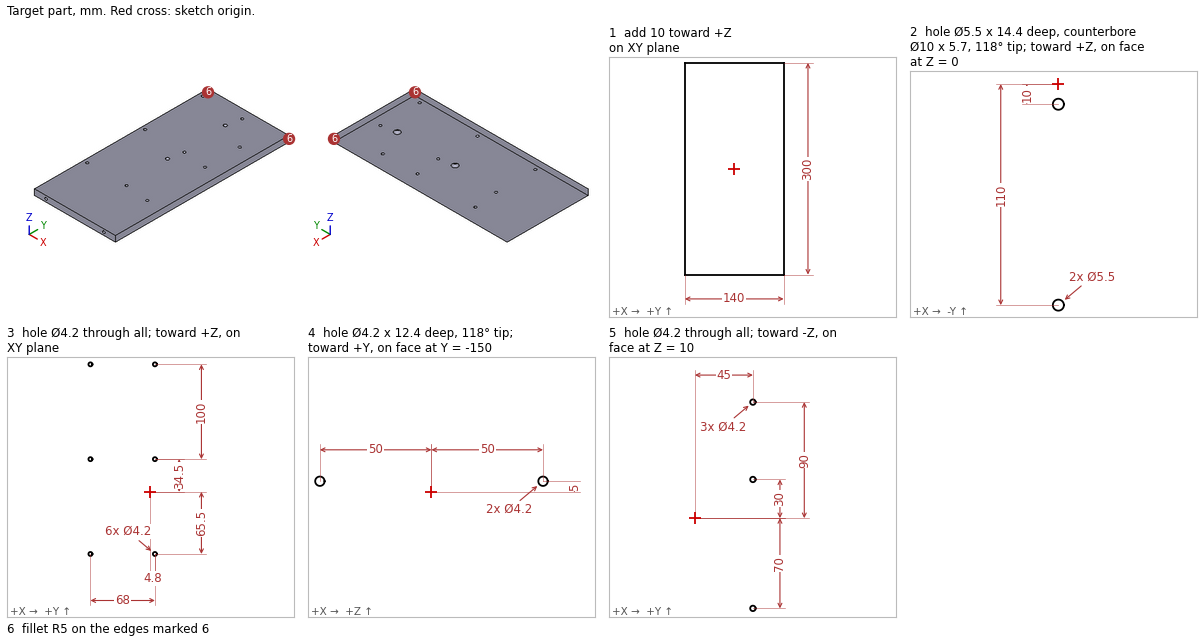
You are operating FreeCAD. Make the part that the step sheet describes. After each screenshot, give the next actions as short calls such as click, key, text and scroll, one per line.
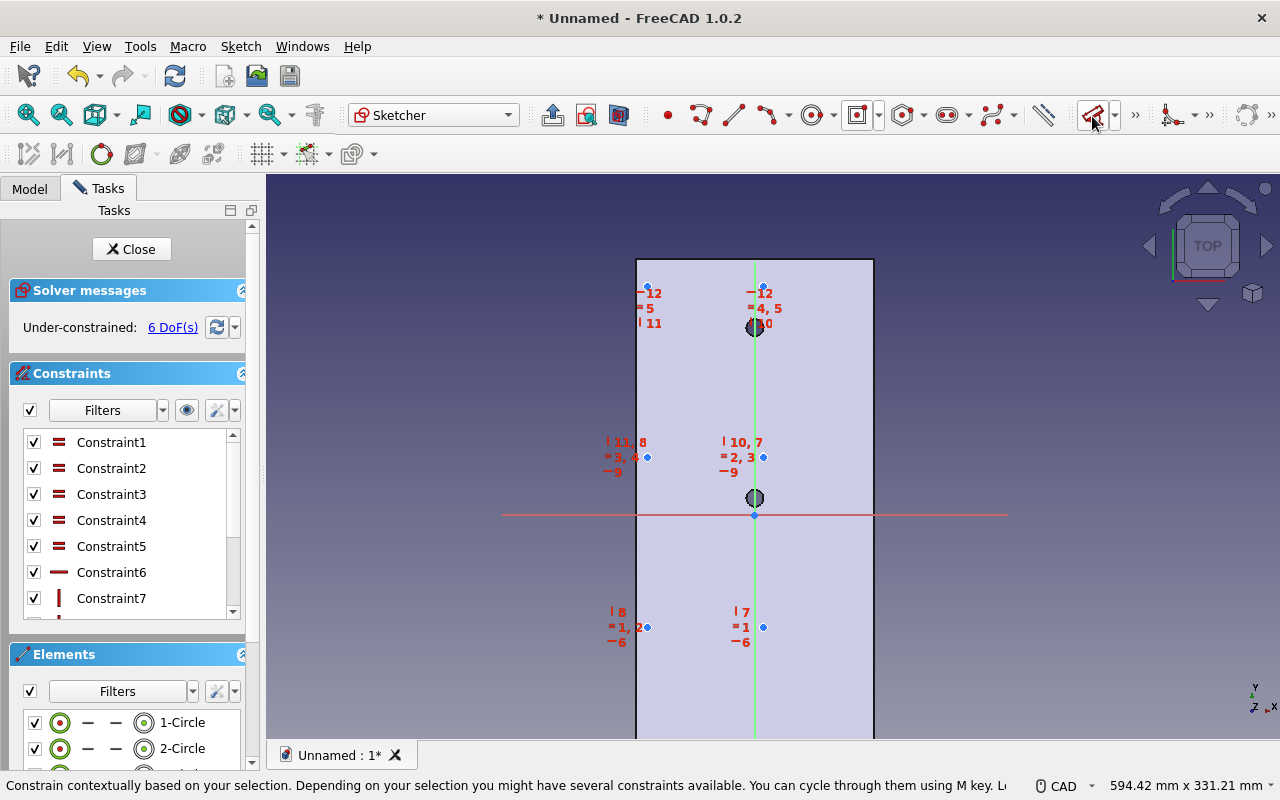
scroll(766, 625, up, 9)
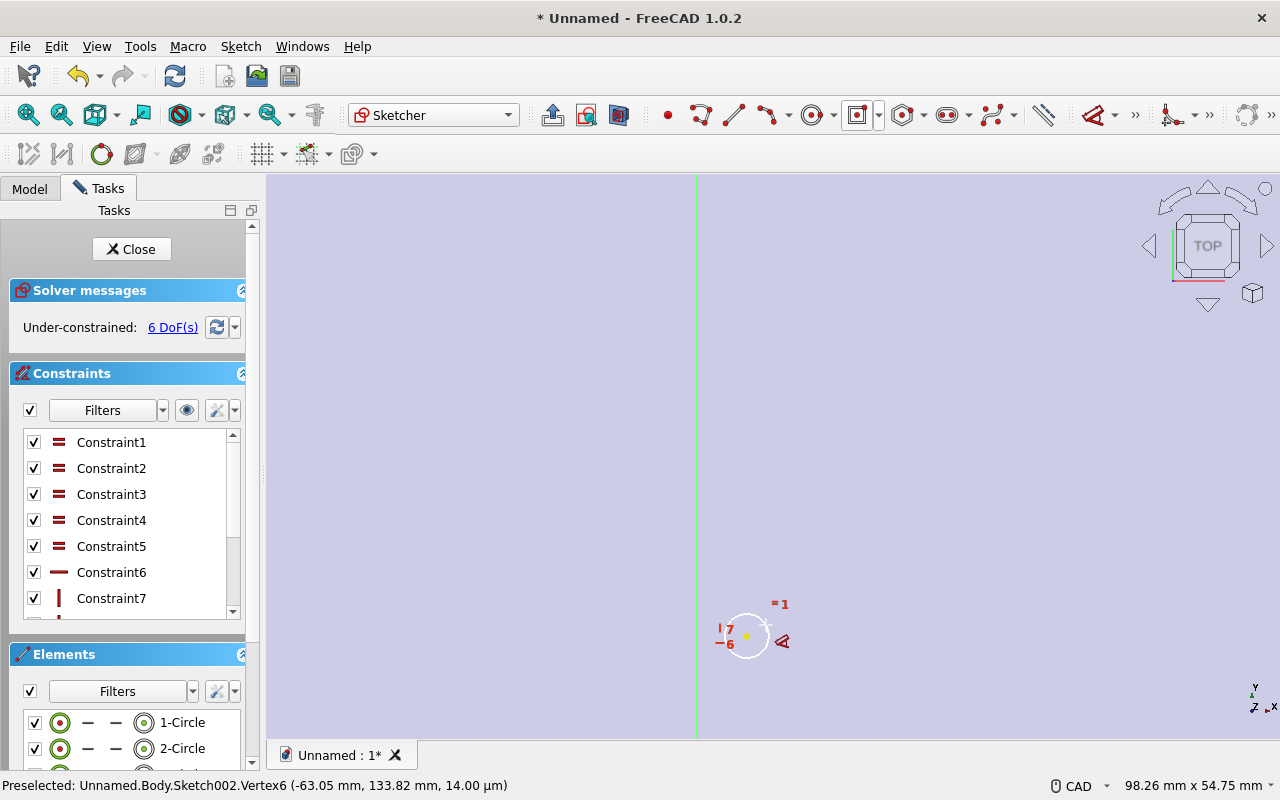
click(762, 620)
click(784, 597)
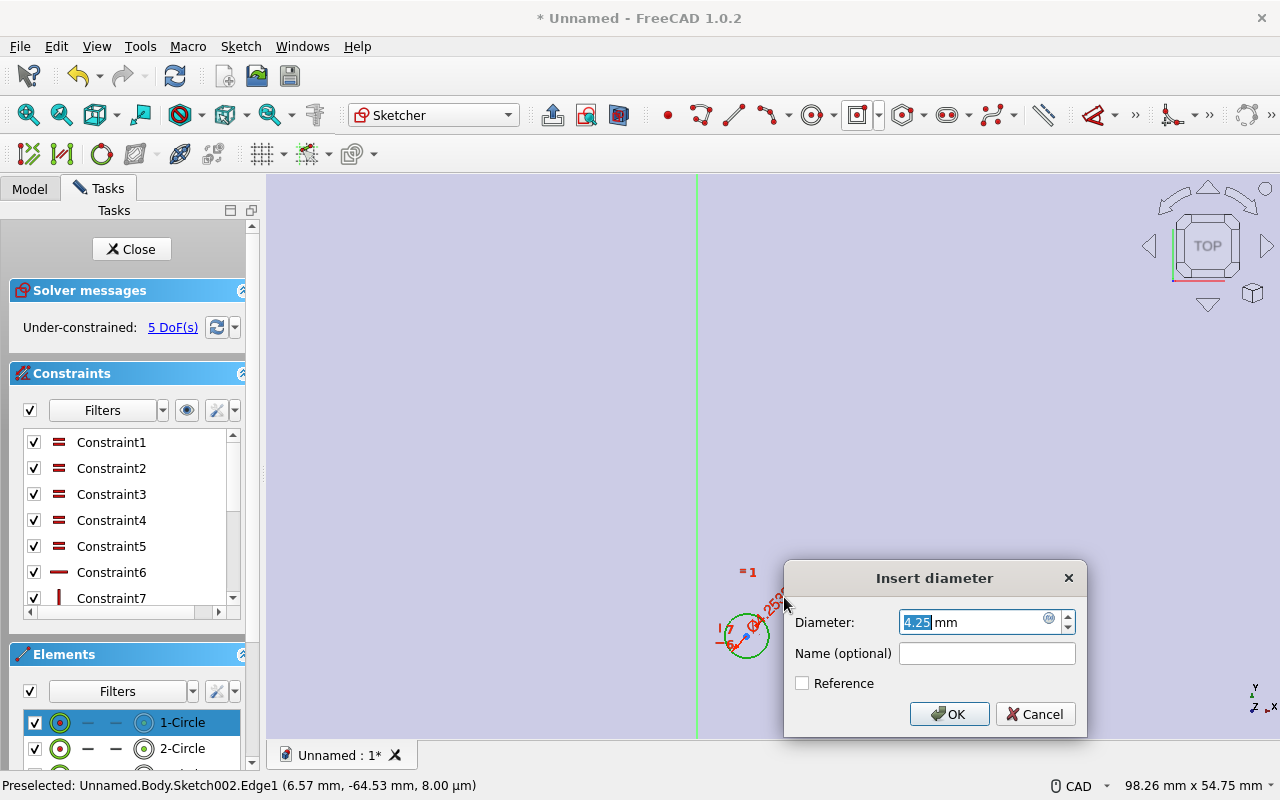
text(4.2)
key(Return)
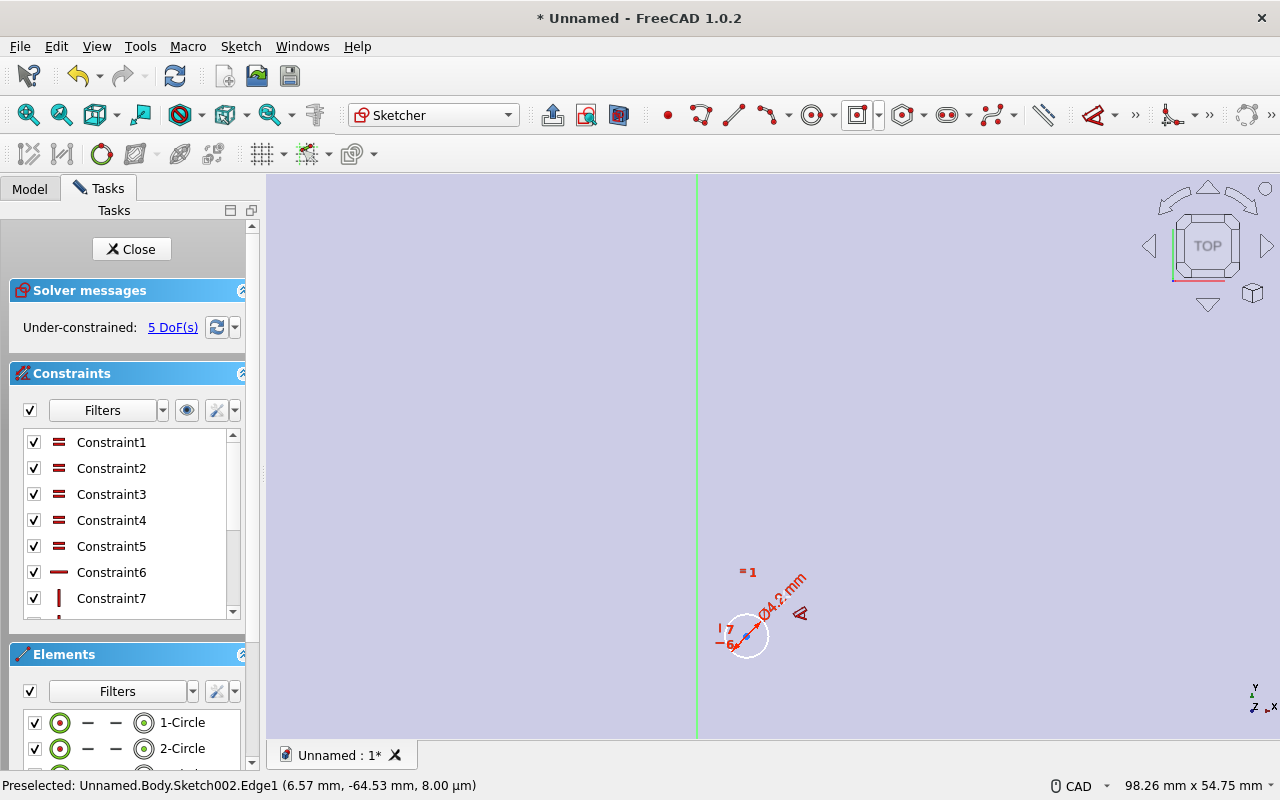
click(747, 636)
click(722, 670)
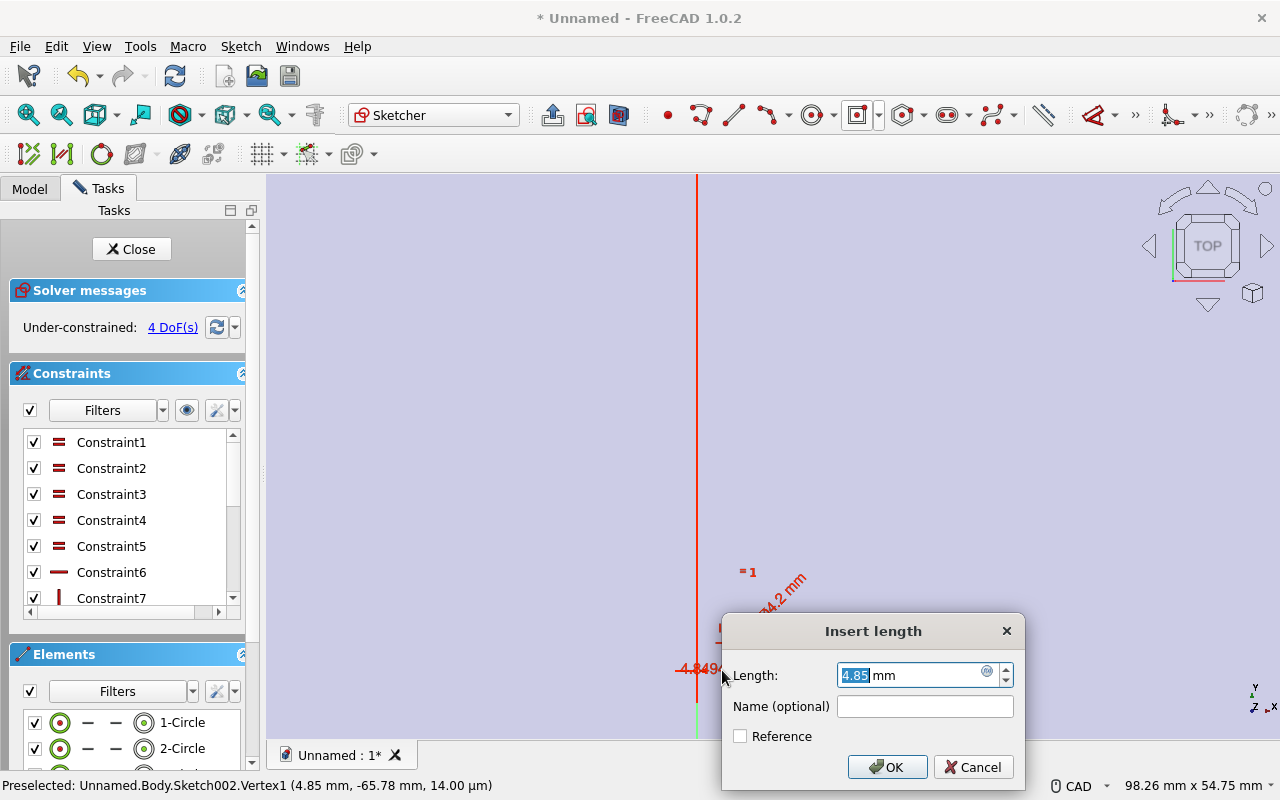
text(4.8)
key(Return)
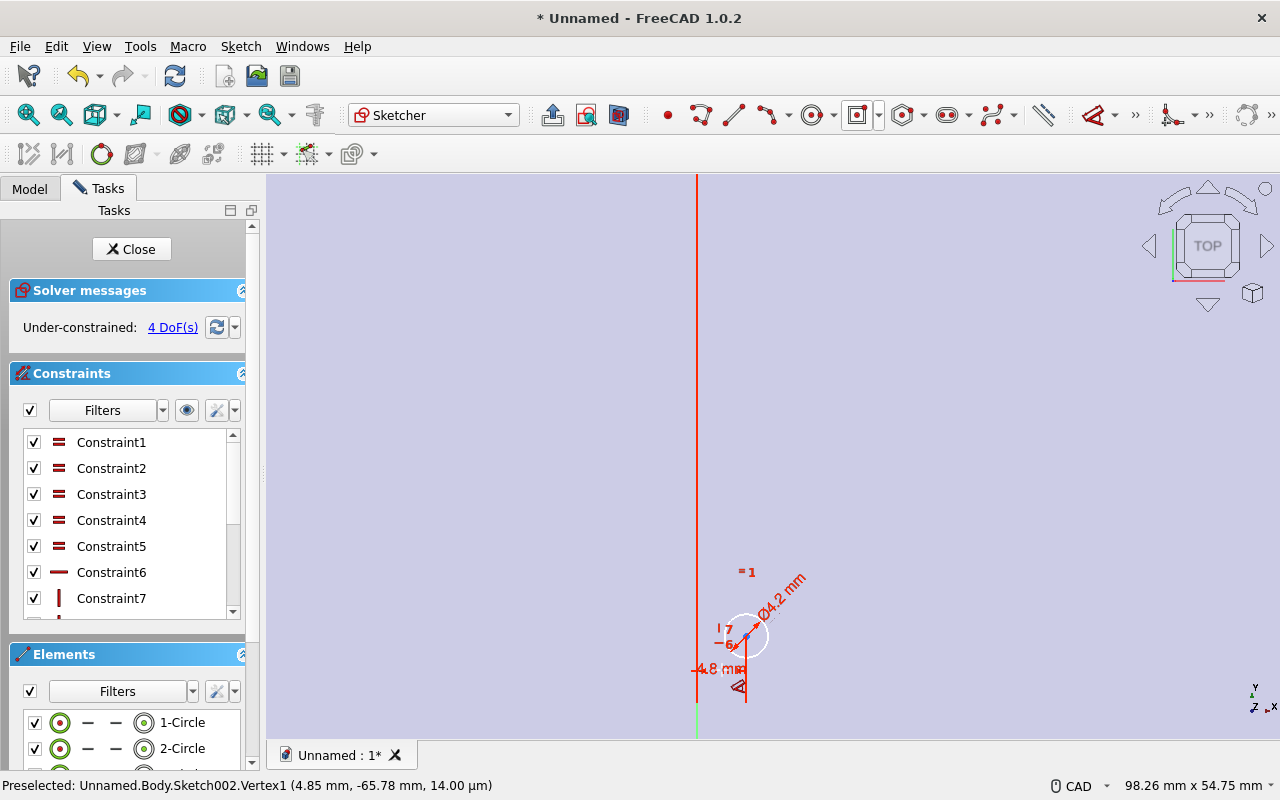
scroll(766, 626, down, 9)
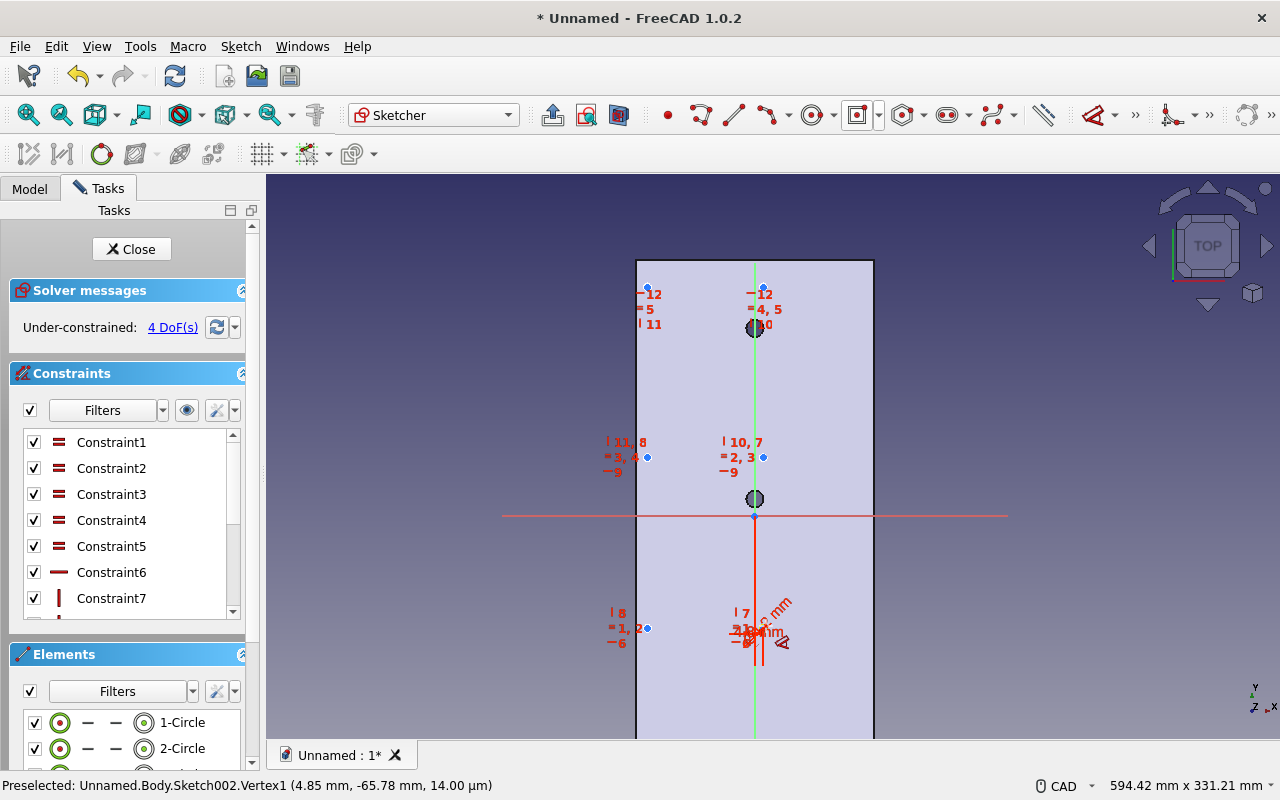
click(763, 628)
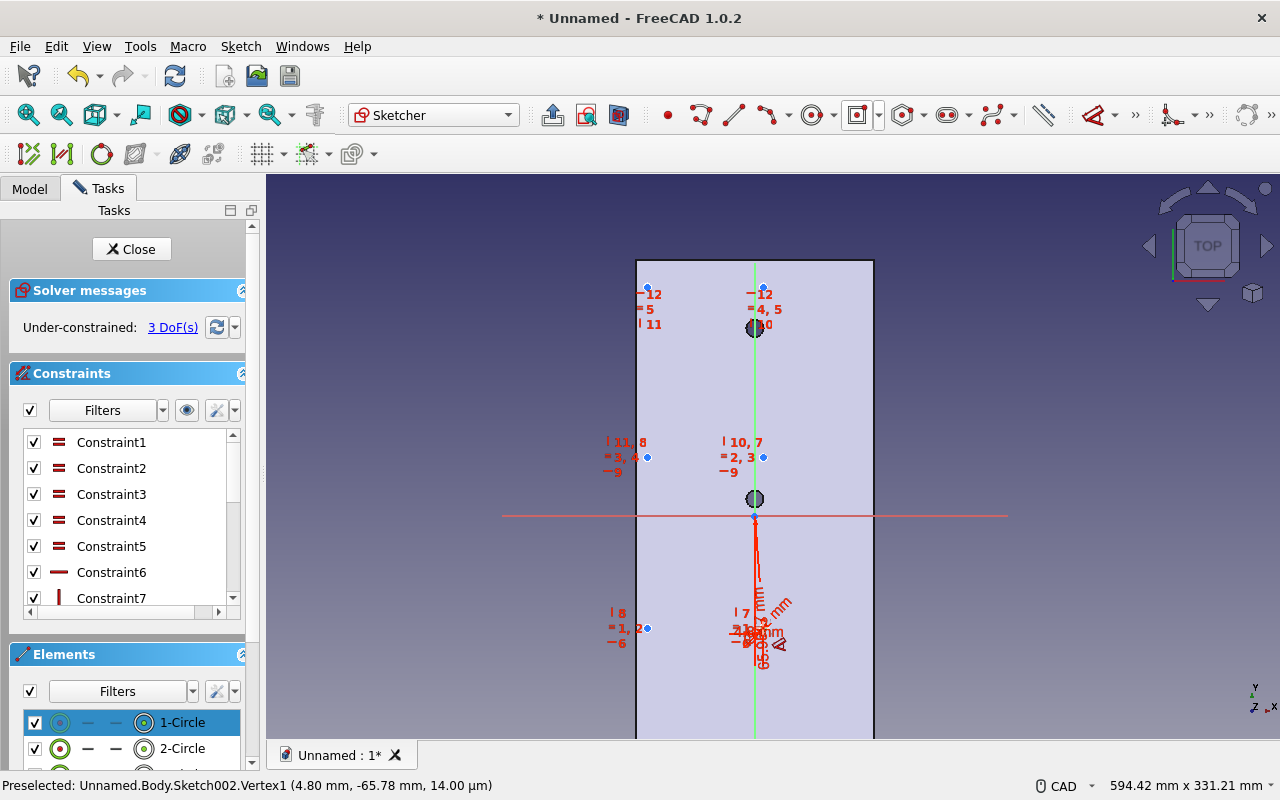
click(647, 628)
click(705, 662)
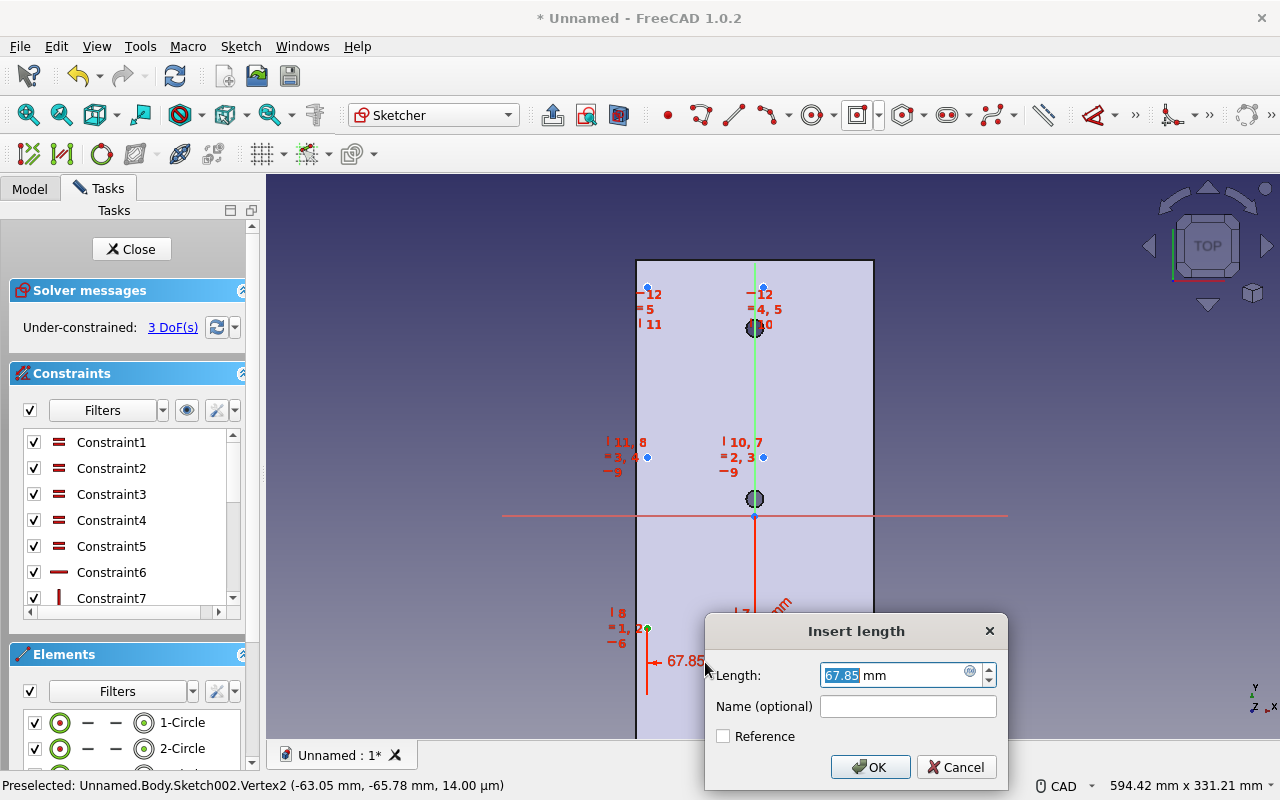
text(68)
key(Return)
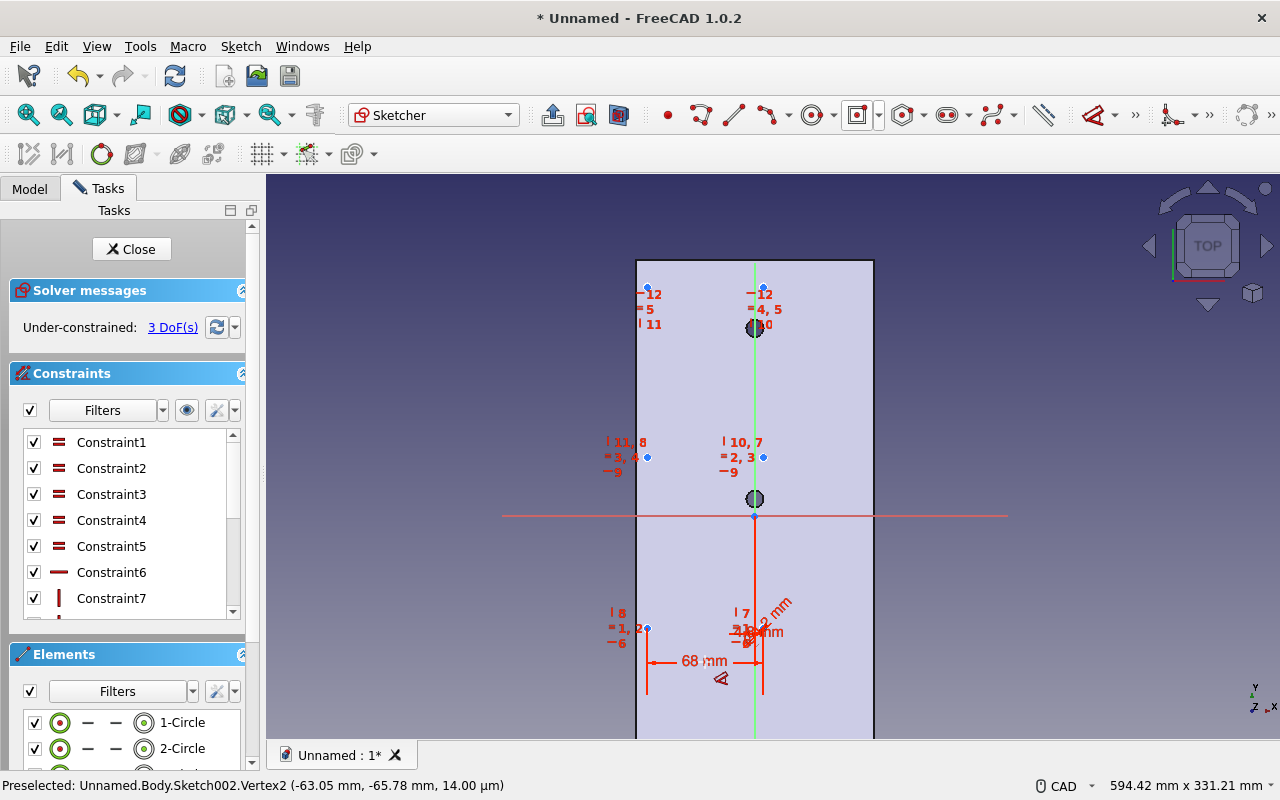
click(763, 628)
click(797, 572)